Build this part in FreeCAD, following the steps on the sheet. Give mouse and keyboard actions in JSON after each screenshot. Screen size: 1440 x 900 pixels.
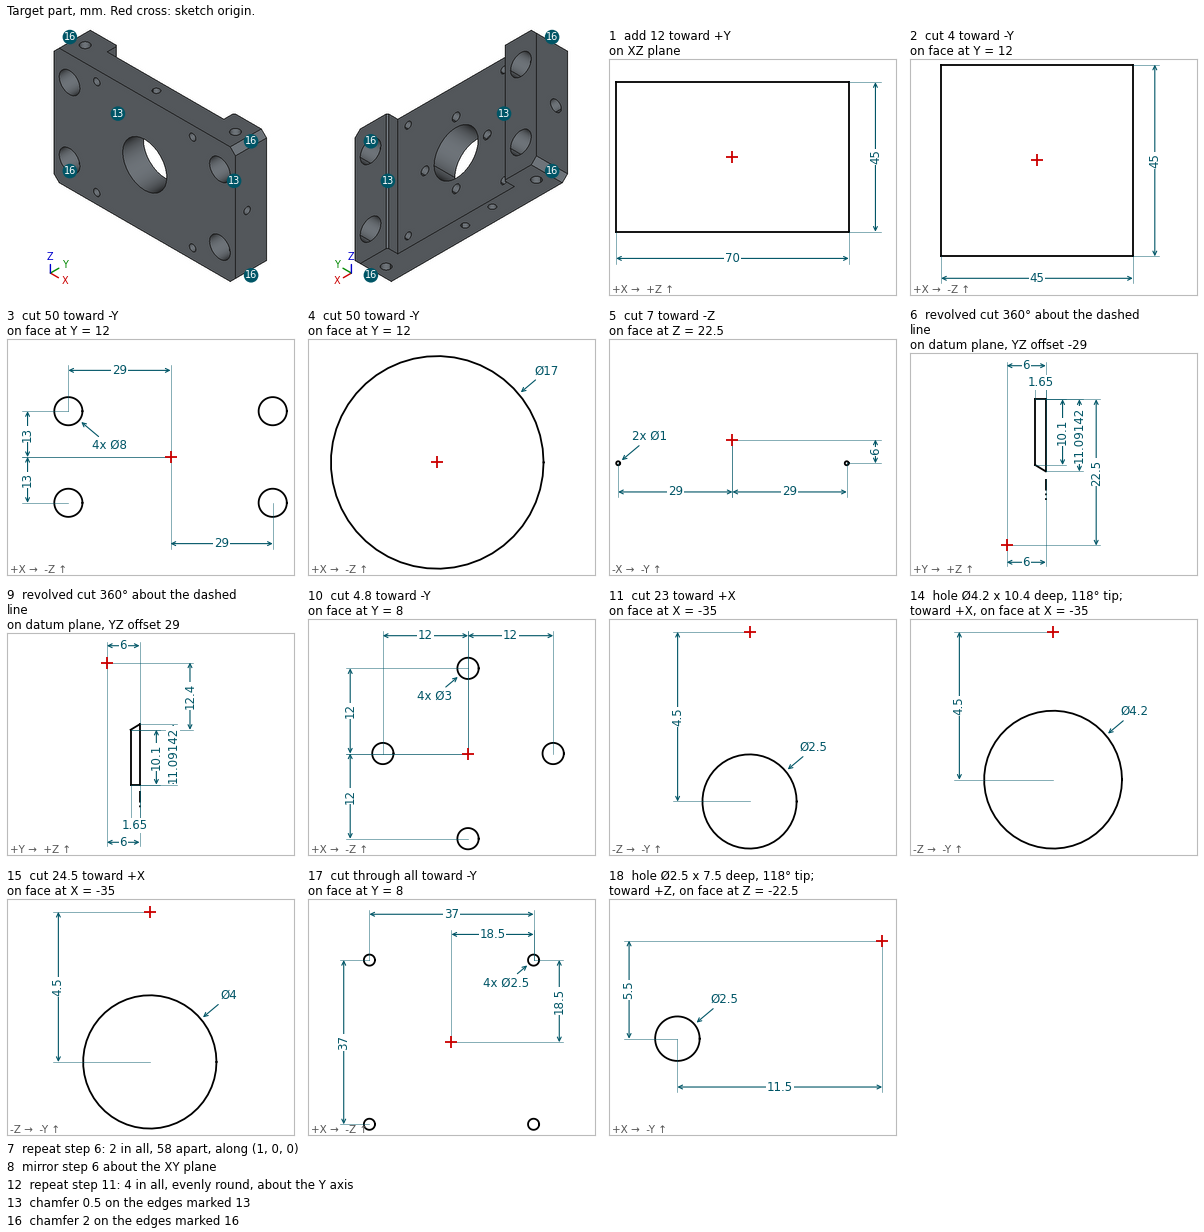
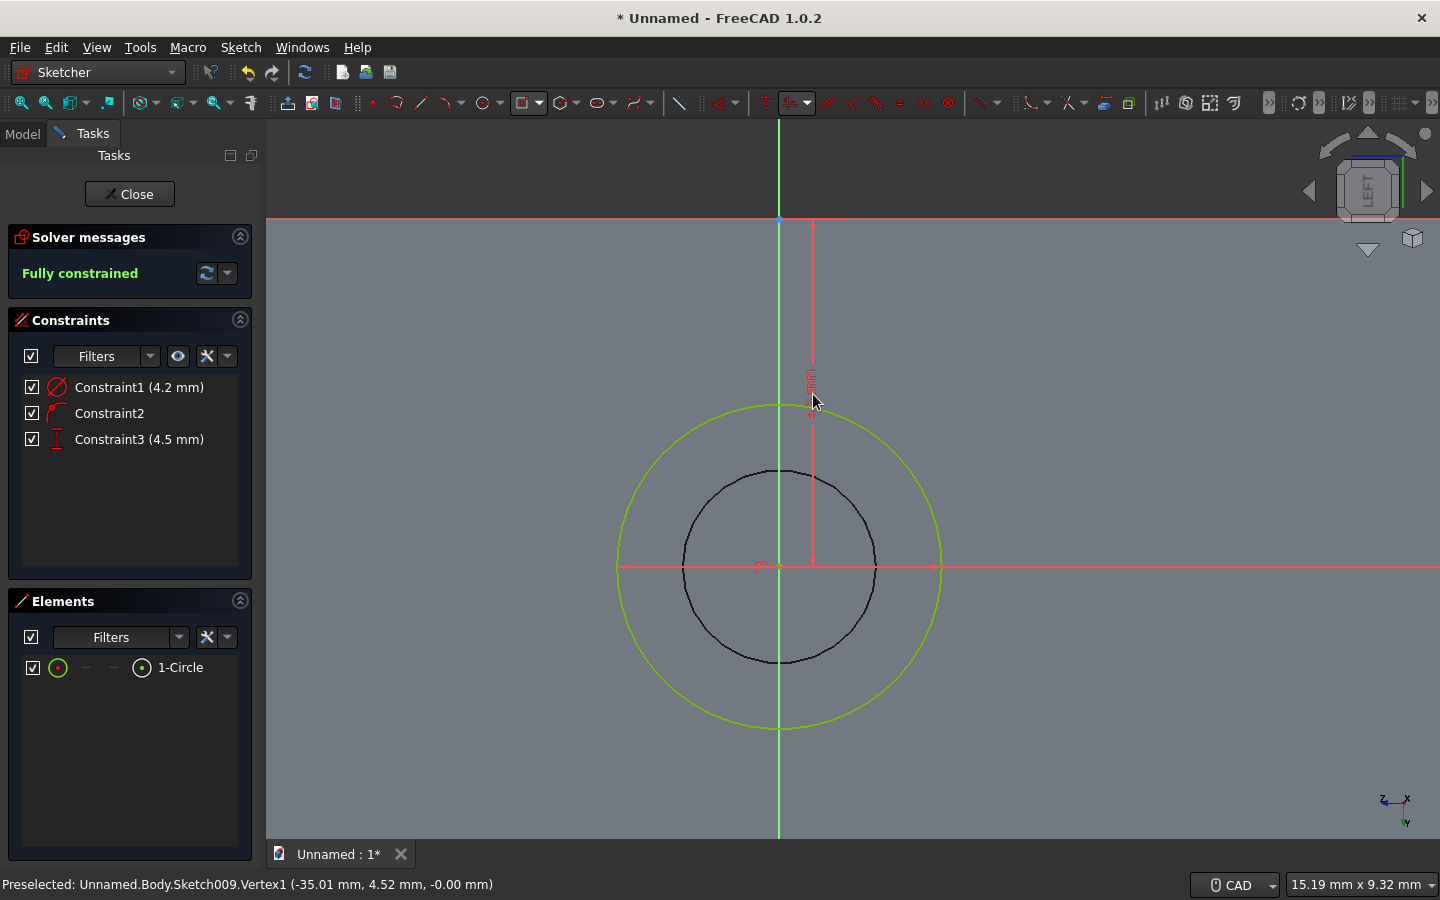
{"action": "left_click", "coordinate": [130, 194]}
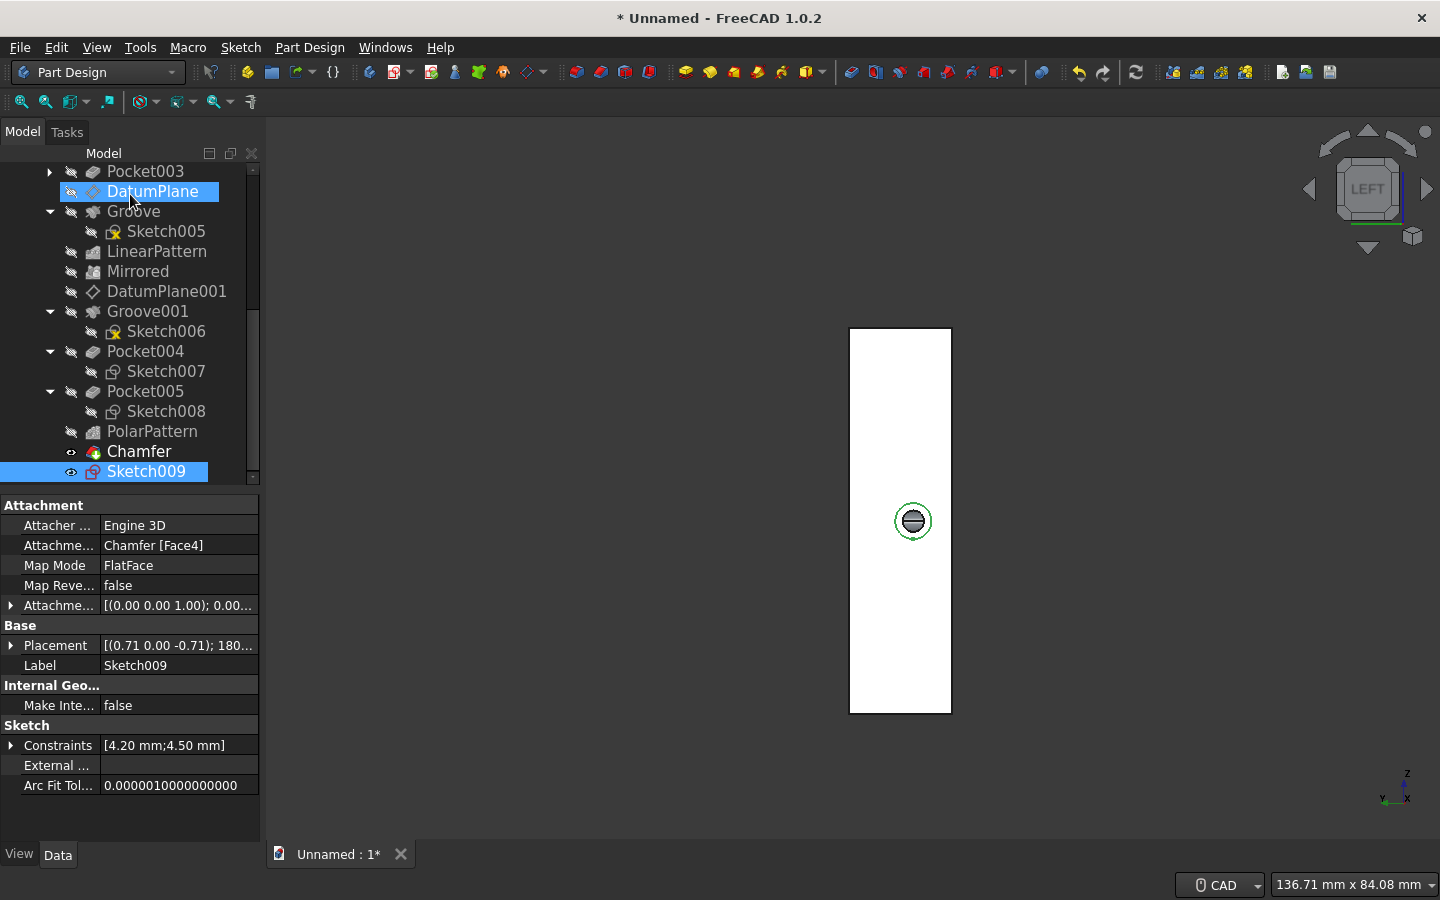
{"action": "left_click", "coordinate": [876, 72]}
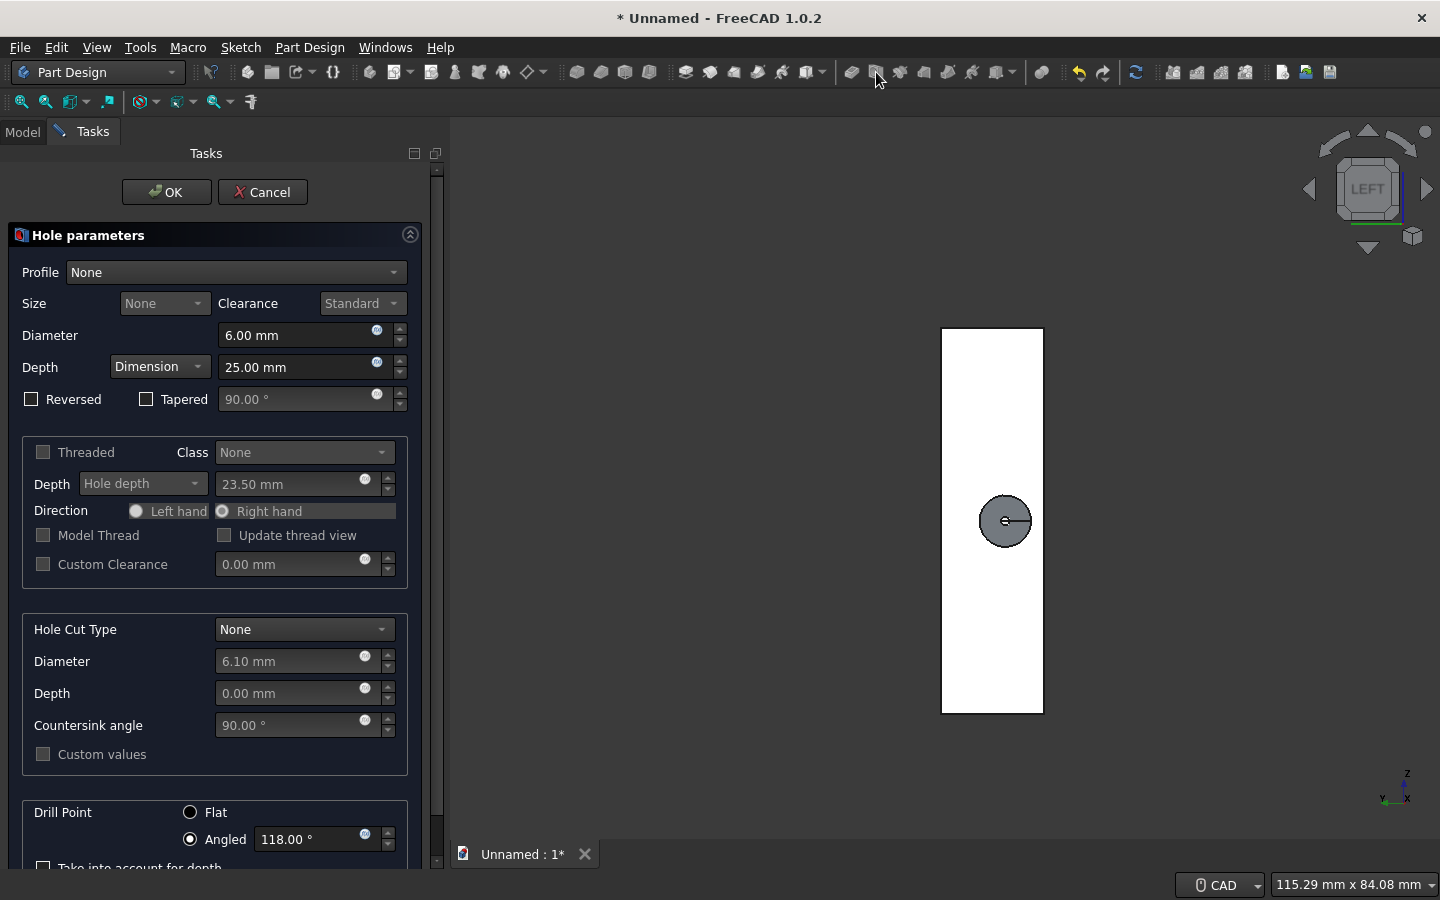
{"action": "triple_click", "coordinate": [305, 335]}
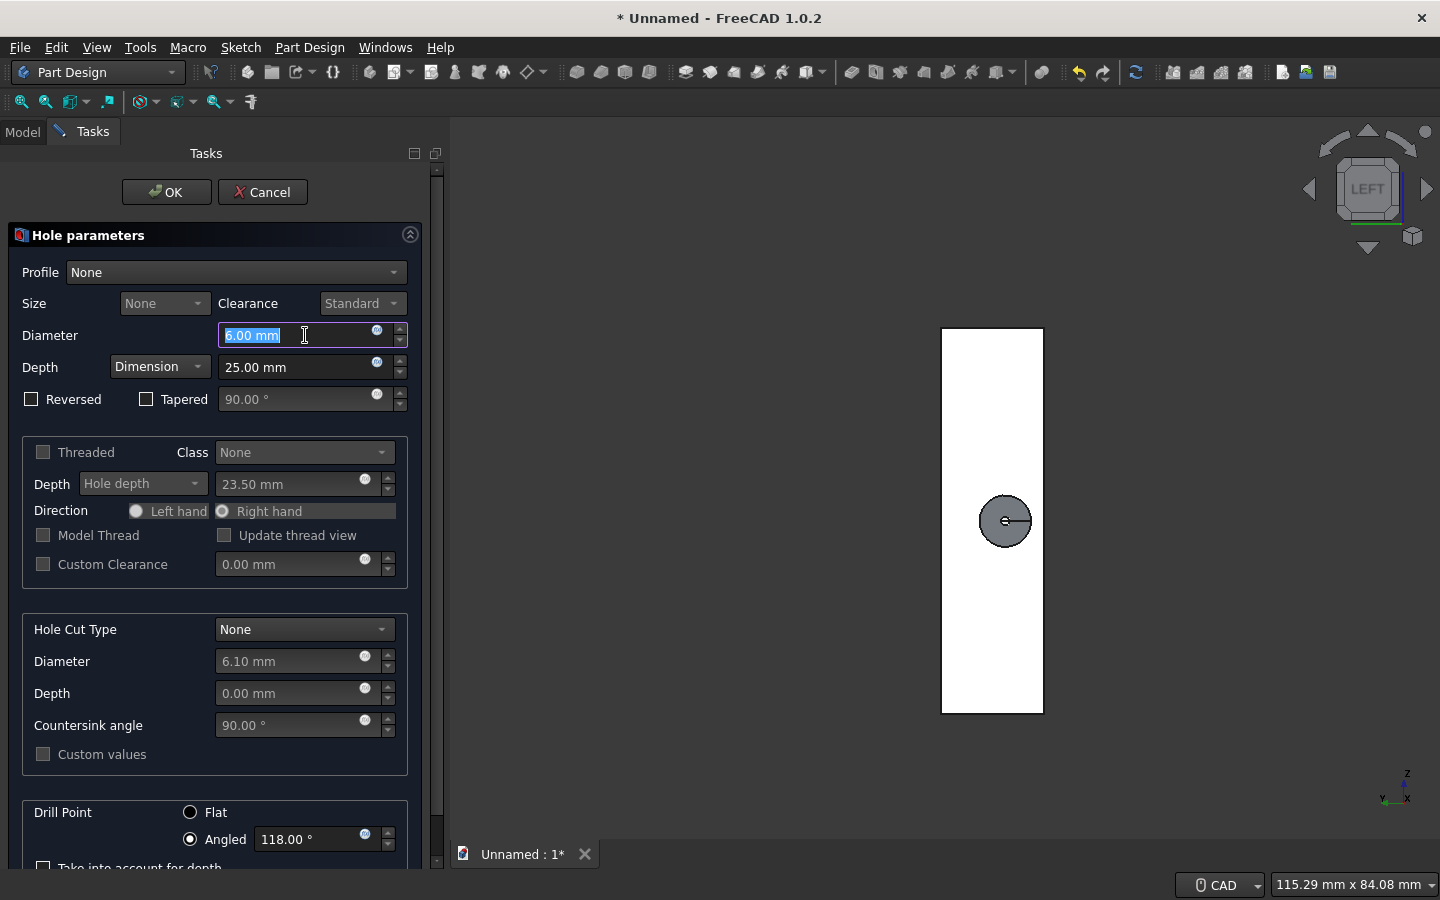
{"action": "type", "text": "4.2"}
{"action": "key", "text": "Tab"}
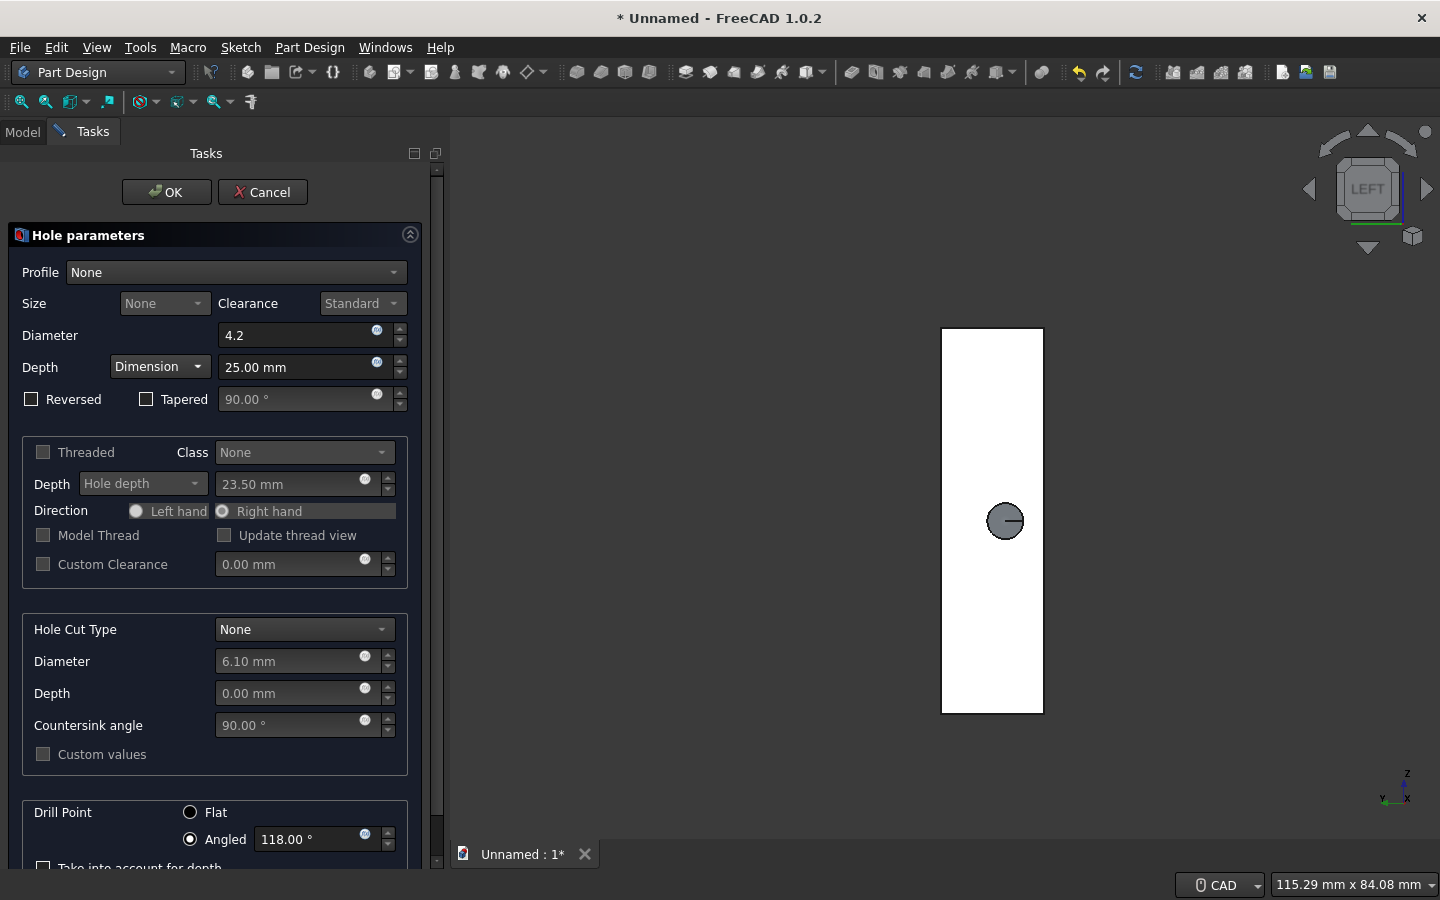
{"action": "triple_click", "coordinate": [305, 367]}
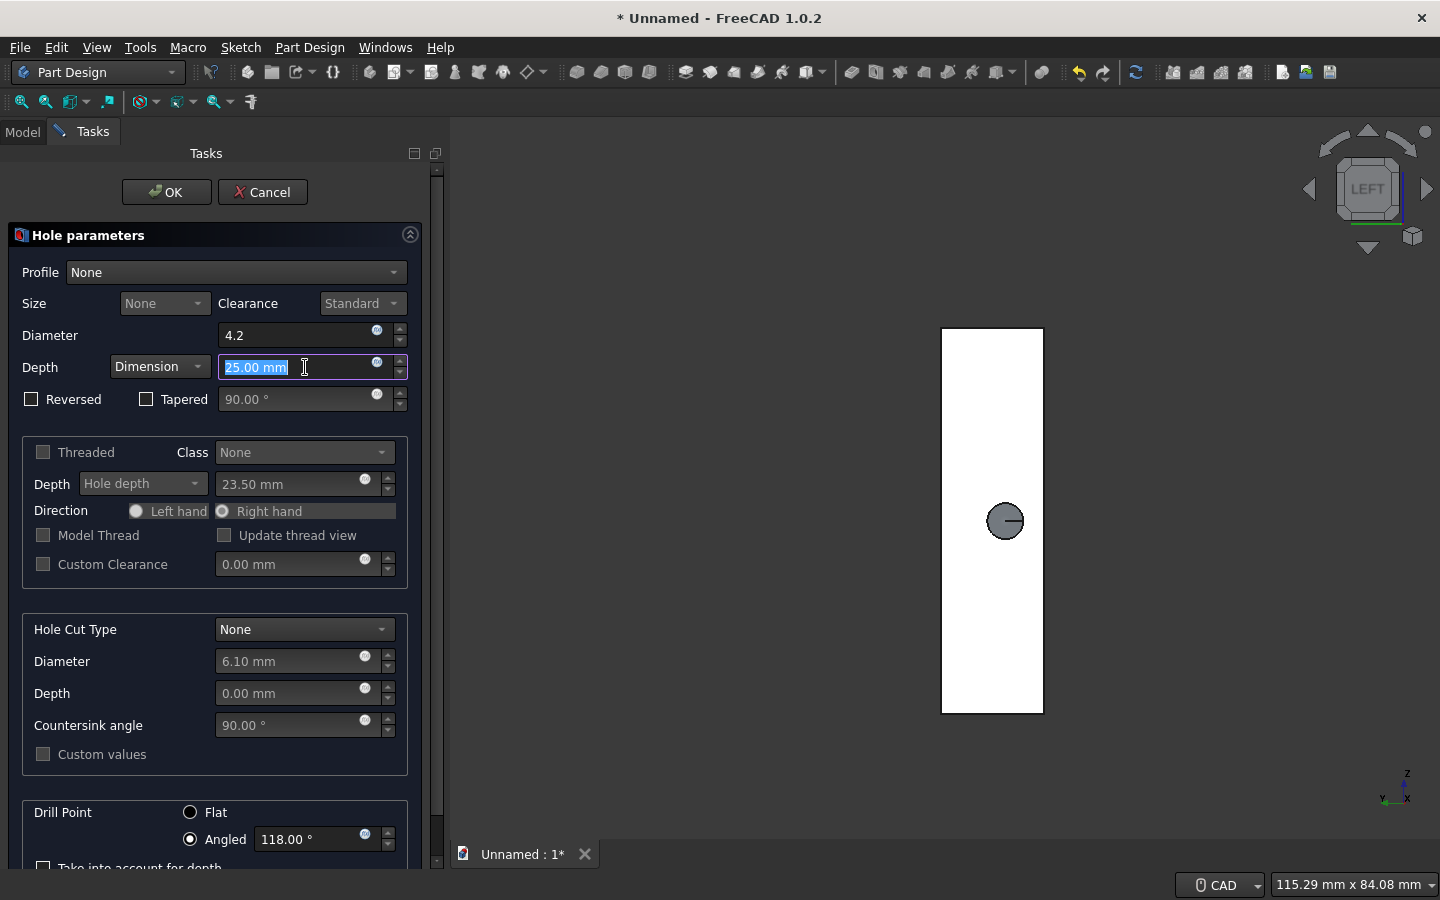
{"action": "type", "text": "10.4"}
{"action": "key", "text": "Tab"}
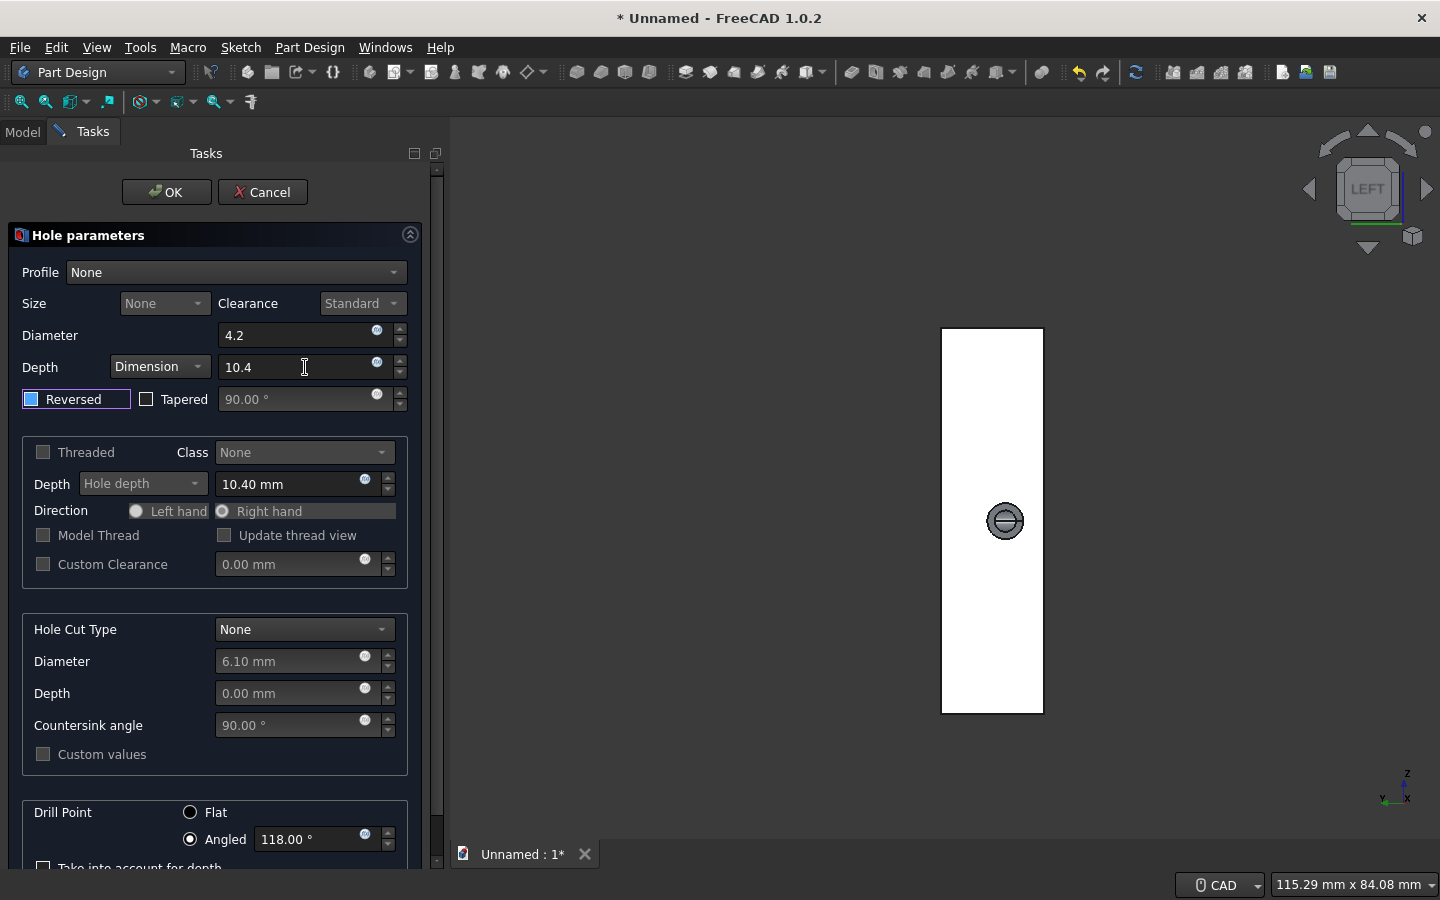
{"action": "left_click", "coordinate": [167, 192]}